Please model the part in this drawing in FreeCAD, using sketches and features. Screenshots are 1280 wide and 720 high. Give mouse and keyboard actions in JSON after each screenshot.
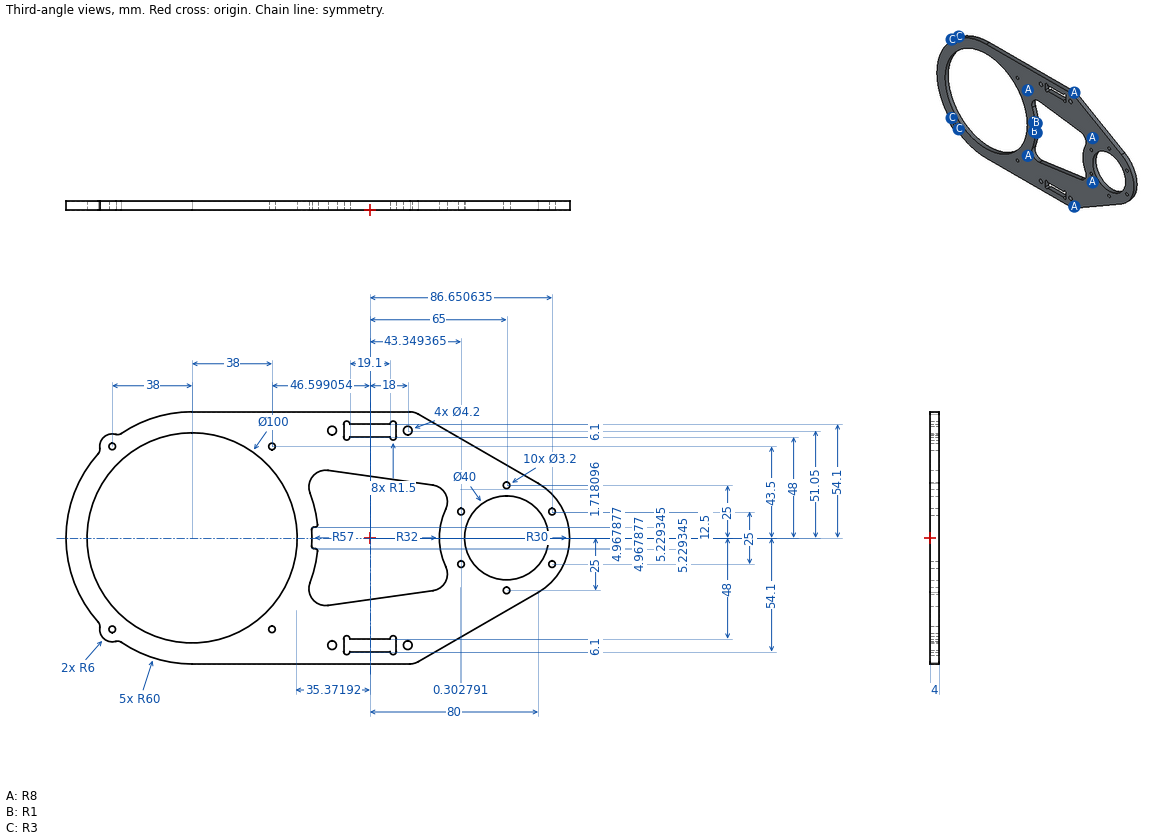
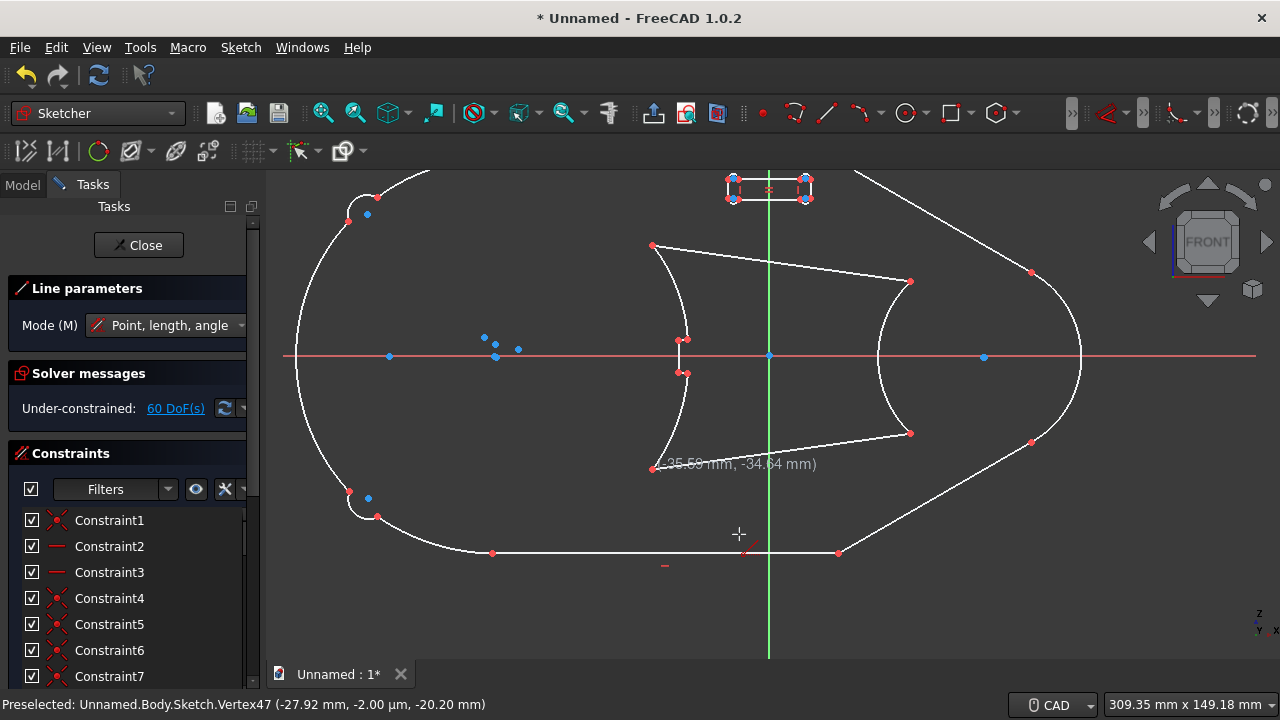
{"action": "left_click", "coordinate": [738, 533]}
{"action": "left_click", "coordinate": [801, 533]}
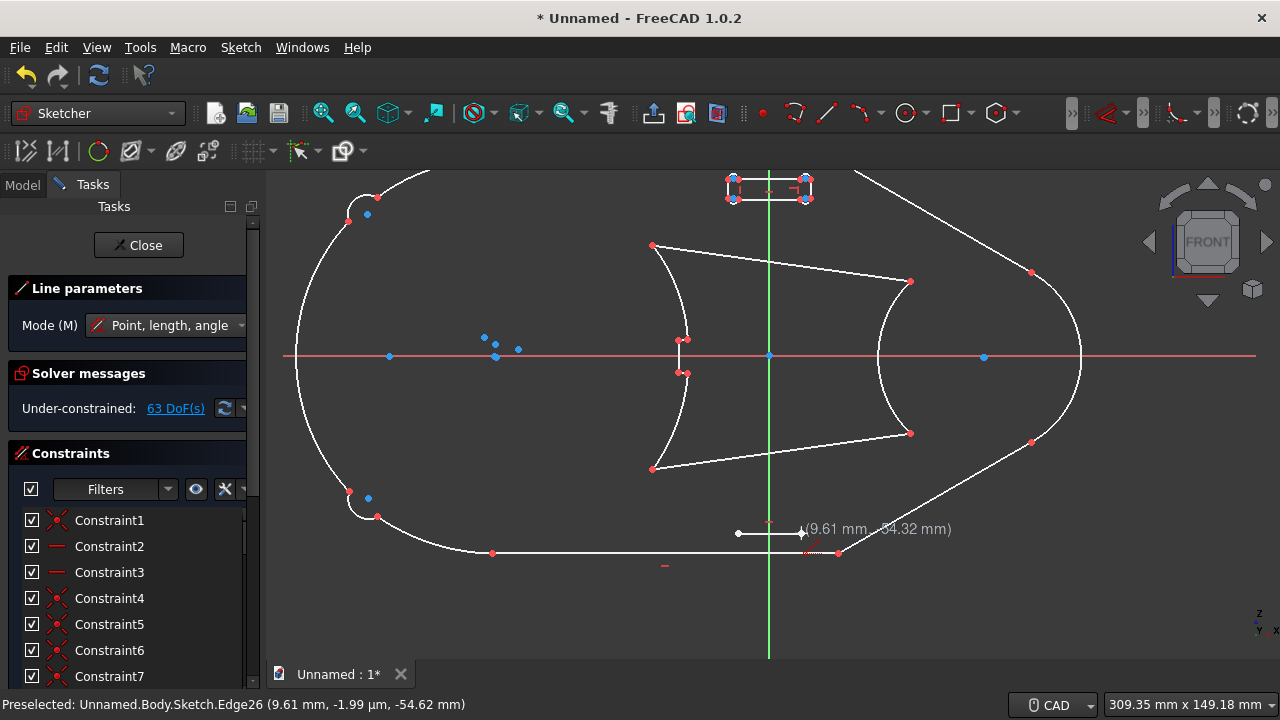
{"action": "scroll", "coordinate": [811, 533], "scroll_direction": "up", "scroll_amount": 3}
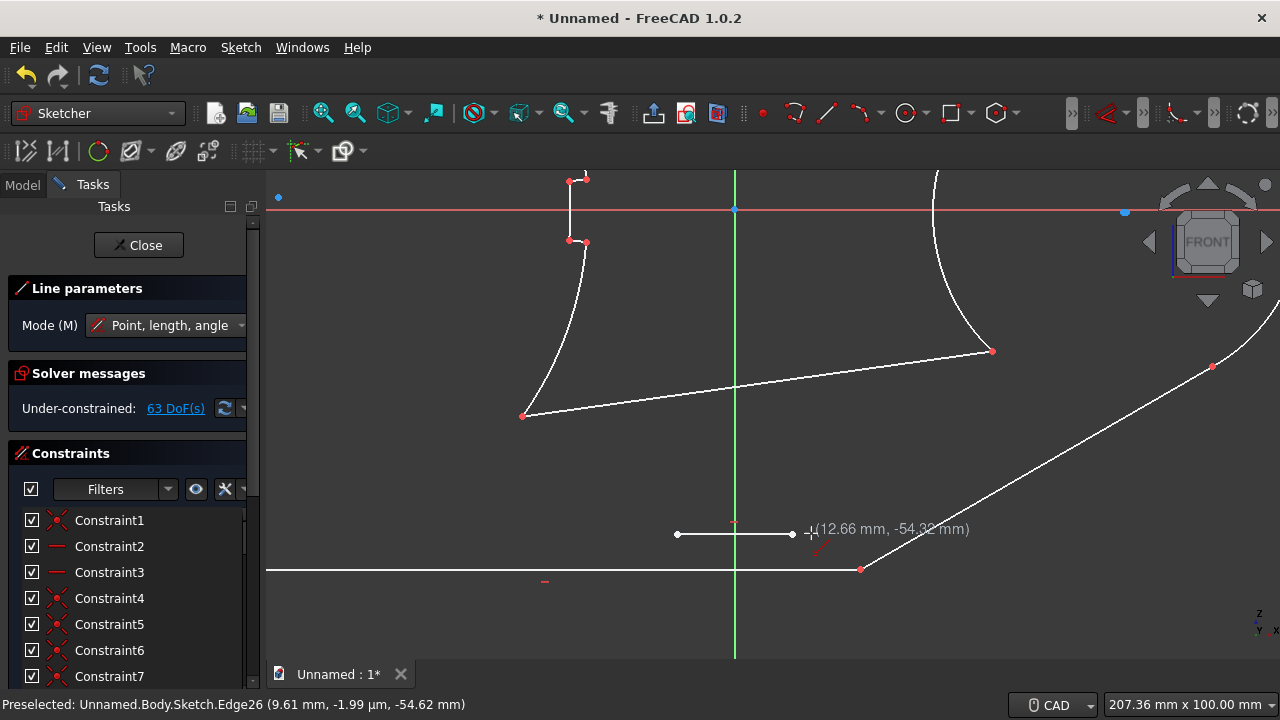
{"action": "left_click", "coordinate": [810, 533]}
{"action": "left_click", "coordinate": [810, 496]}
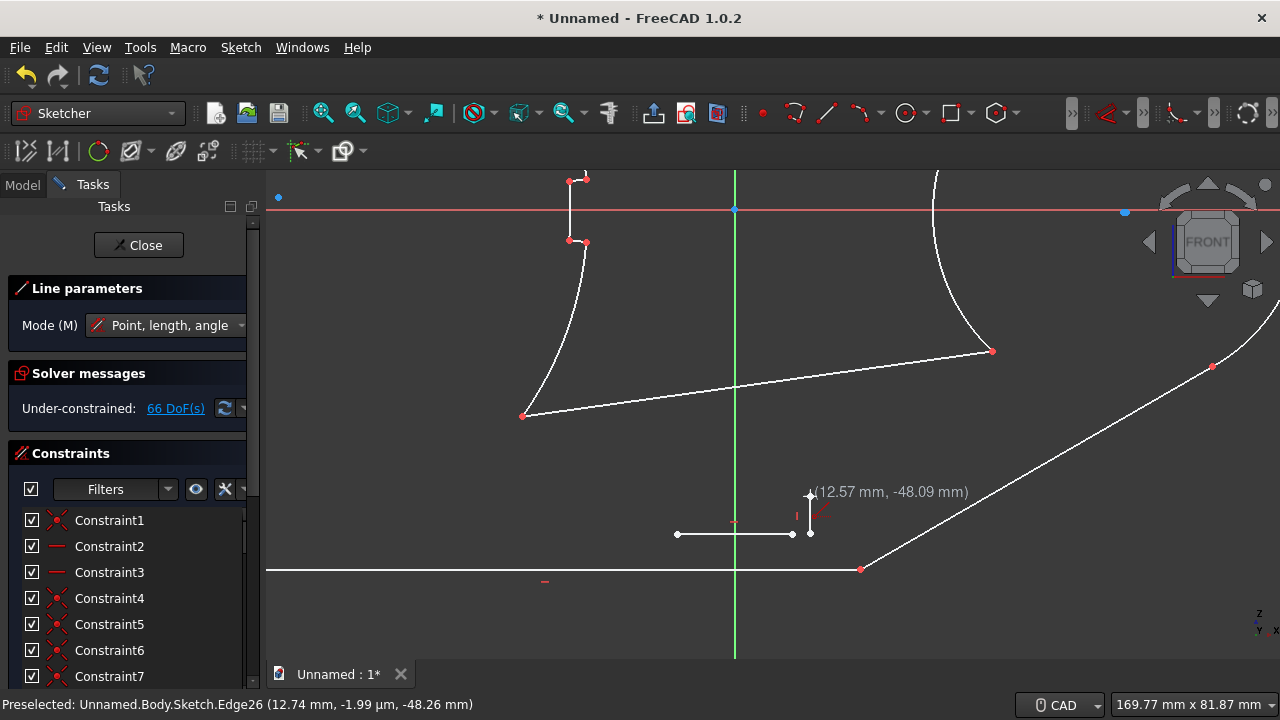
{"action": "left_click", "coordinate": [792, 496]}
{"action": "left_click", "coordinate": [678, 496]}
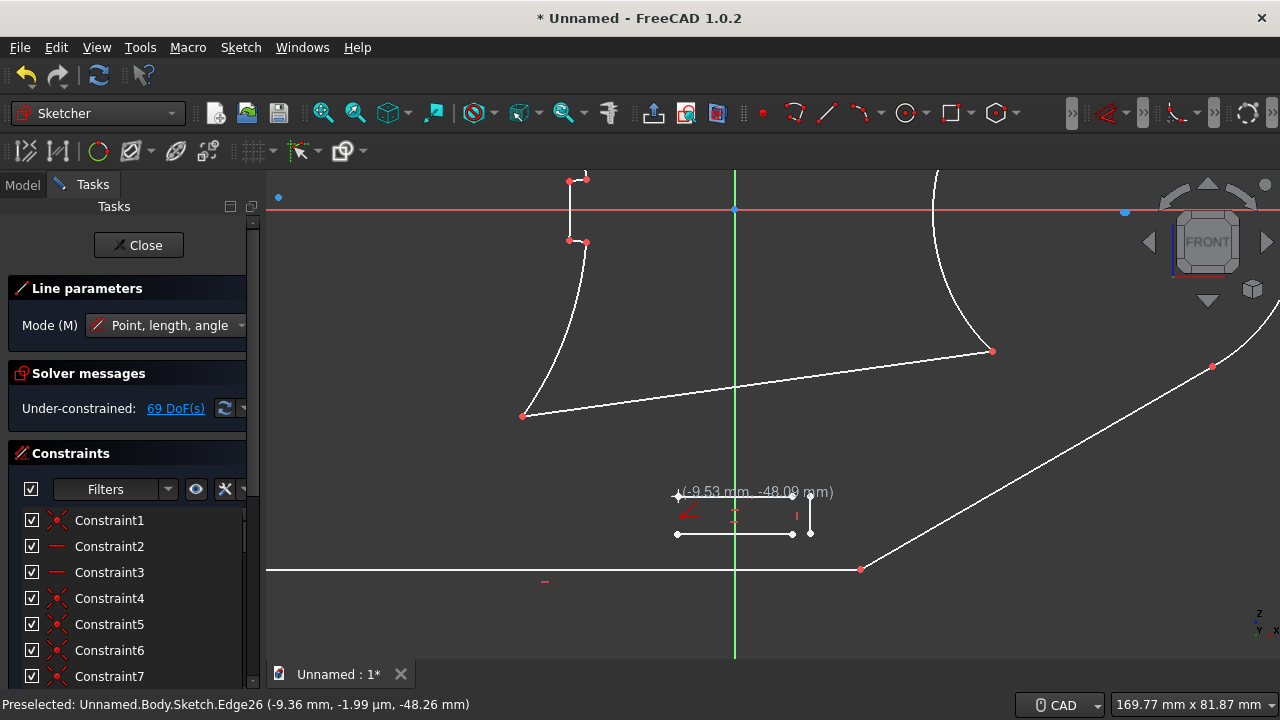
{"action": "left_click", "coordinate": [660, 496]}
{"action": "left_click", "coordinate": [660, 533]}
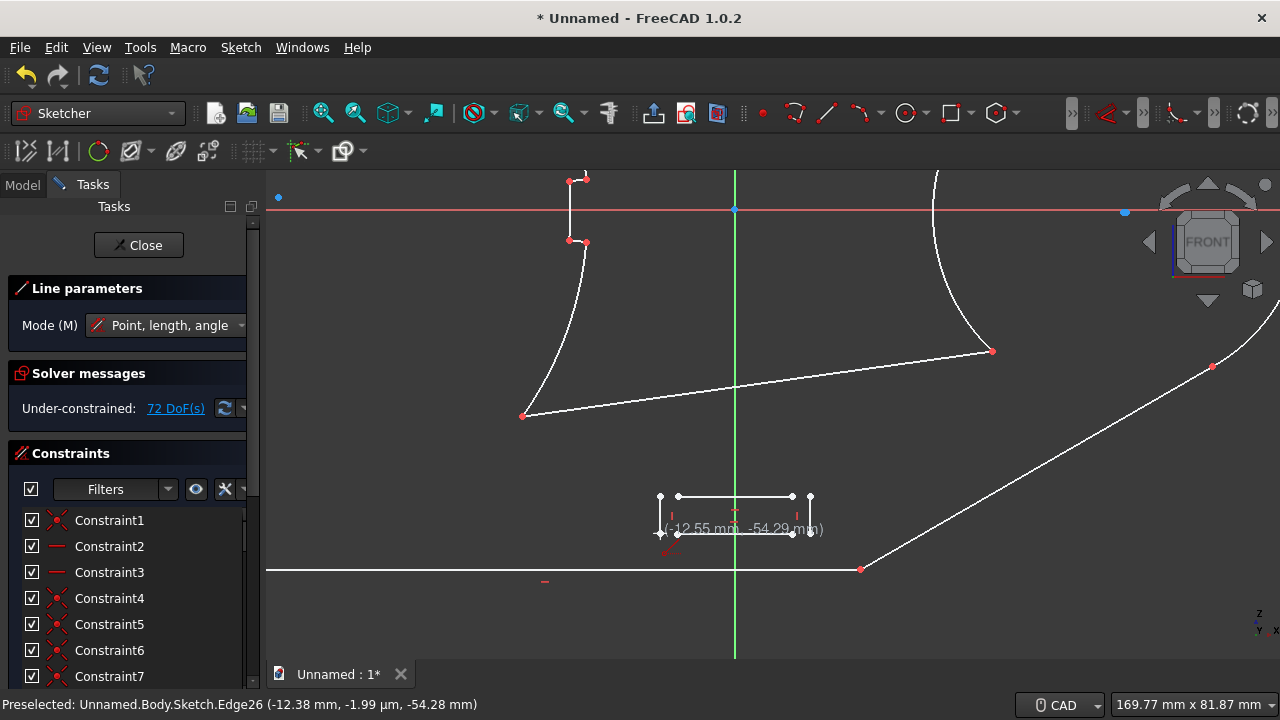
{"action": "left_click", "coordinate": [860, 114]}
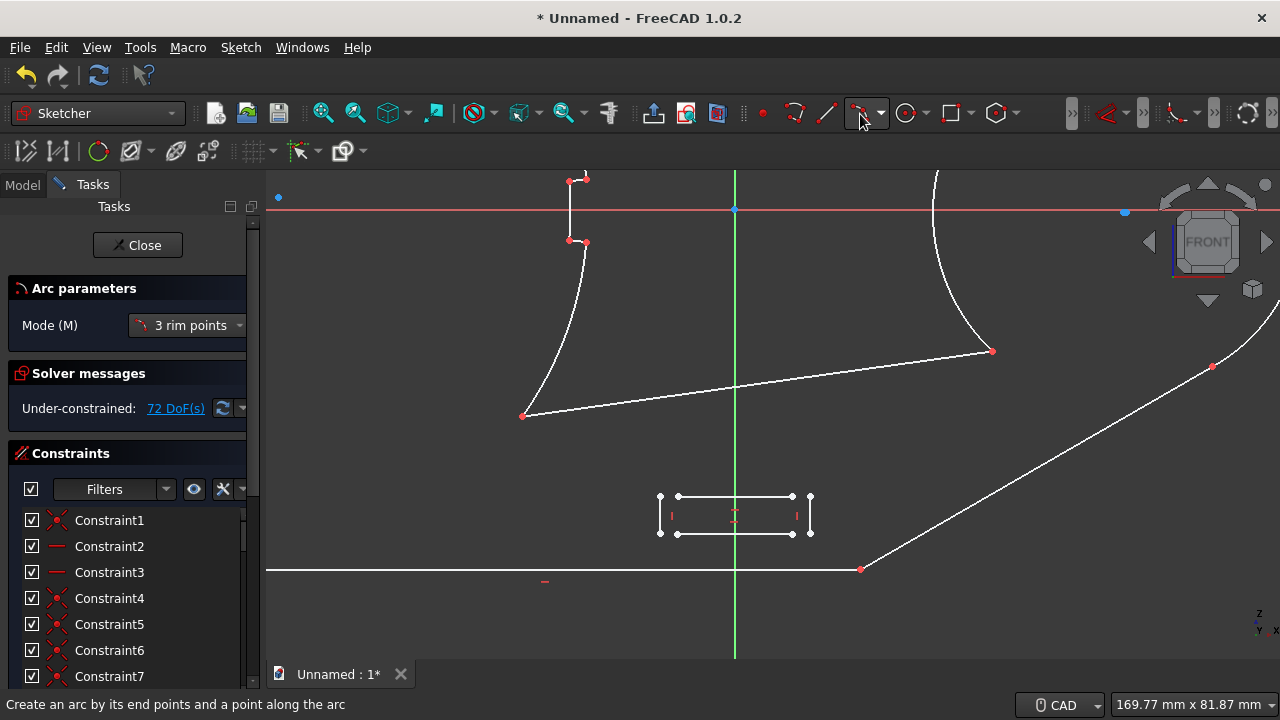
{"action": "left_click", "coordinate": [792, 534]}
{"action": "left_click", "coordinate": [810, 534]}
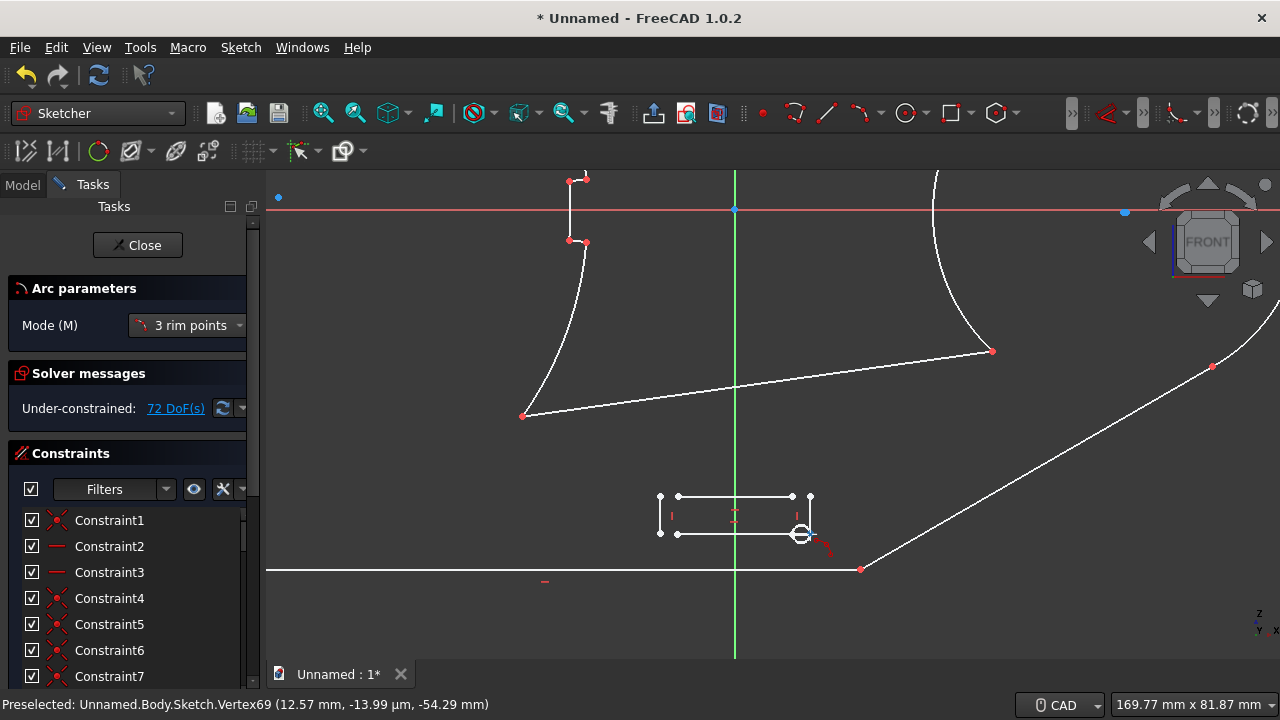
{"action": "scroll", "coordinate": [801, 542], "scroll_direction": "up", "scroll_amount": 3}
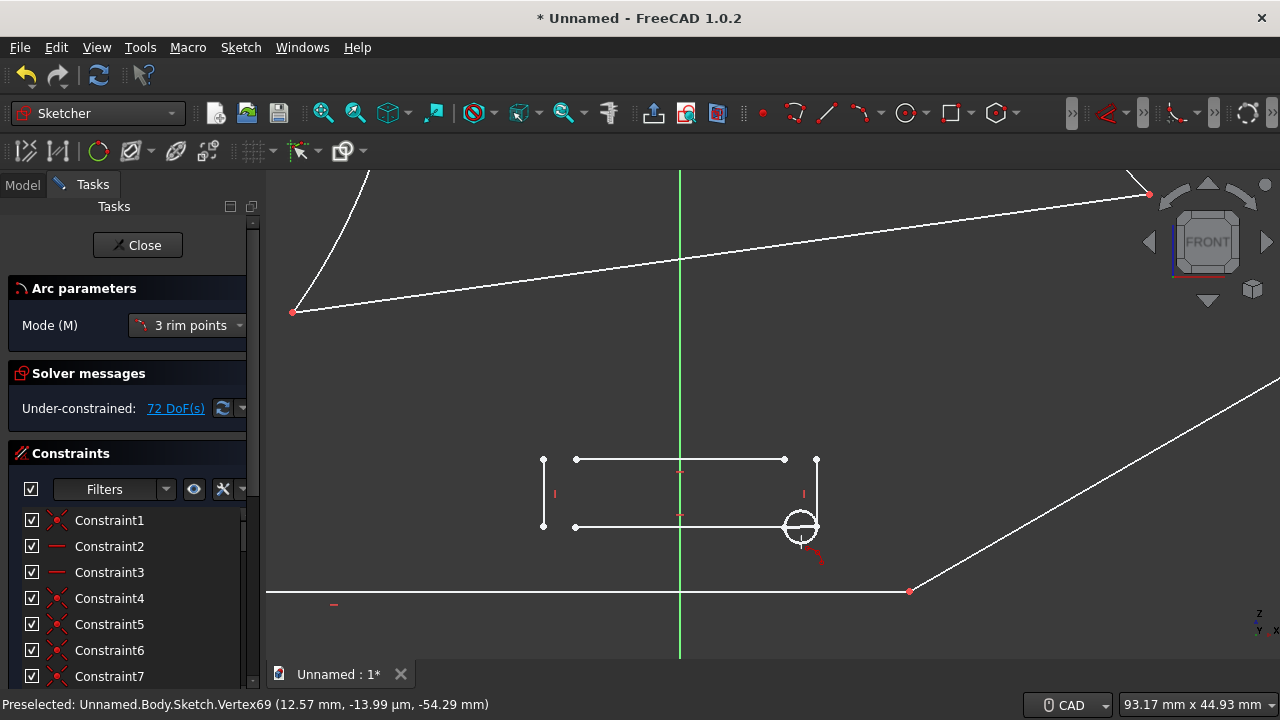
{"action": "left_click", "coordinate": [800, 541]}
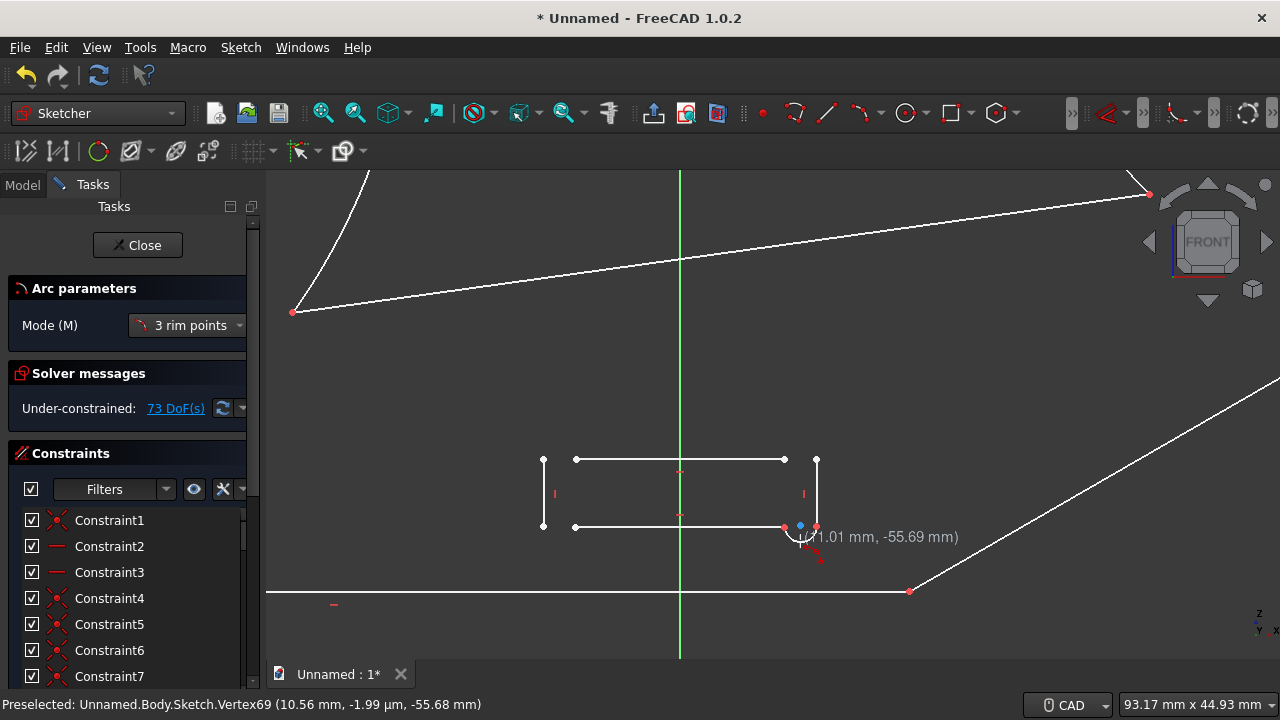
{"action": "left_click", "coordinate": [817, 459]}
{"action": "left_click", "coordinate": [784, 459]}
{"action": "left_click", "coordinate": [800, 442]}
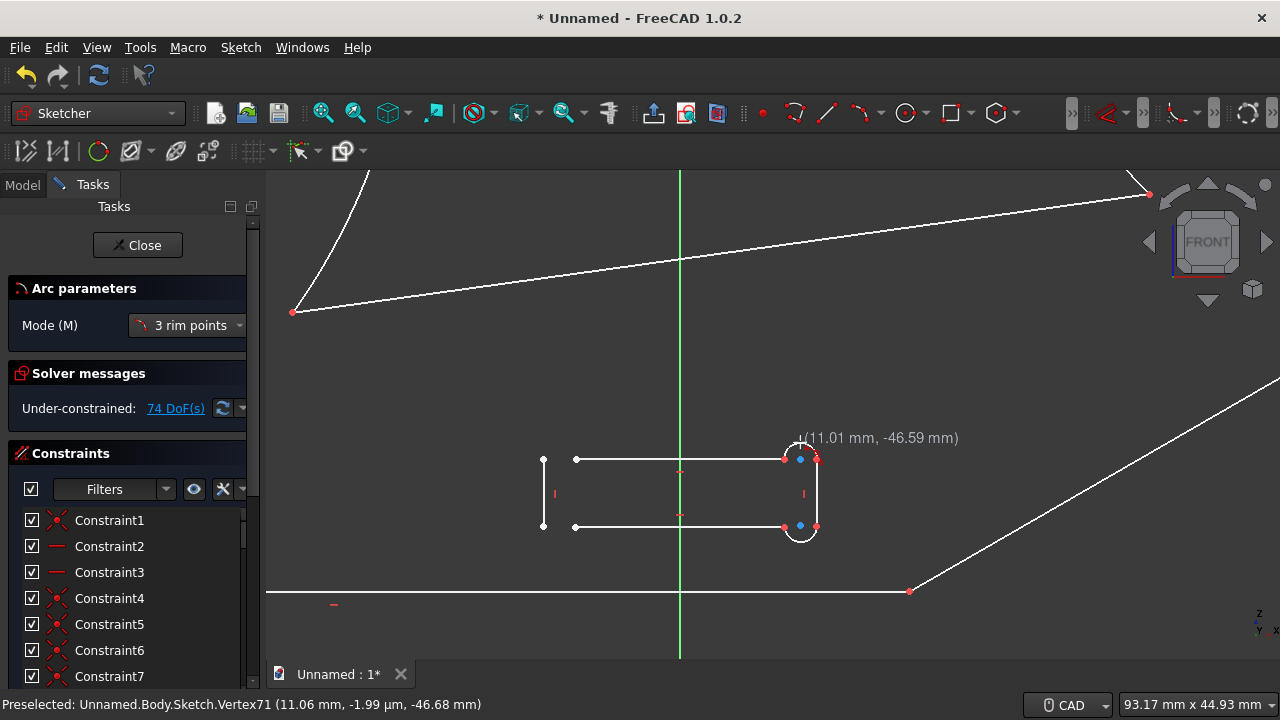
{"action": "left_click", "coordinate": [576, 459]}
{"action": "left_click", "coordinate": [544, 459]}
{"action": "left_click", "coordinate": [560, 442]}